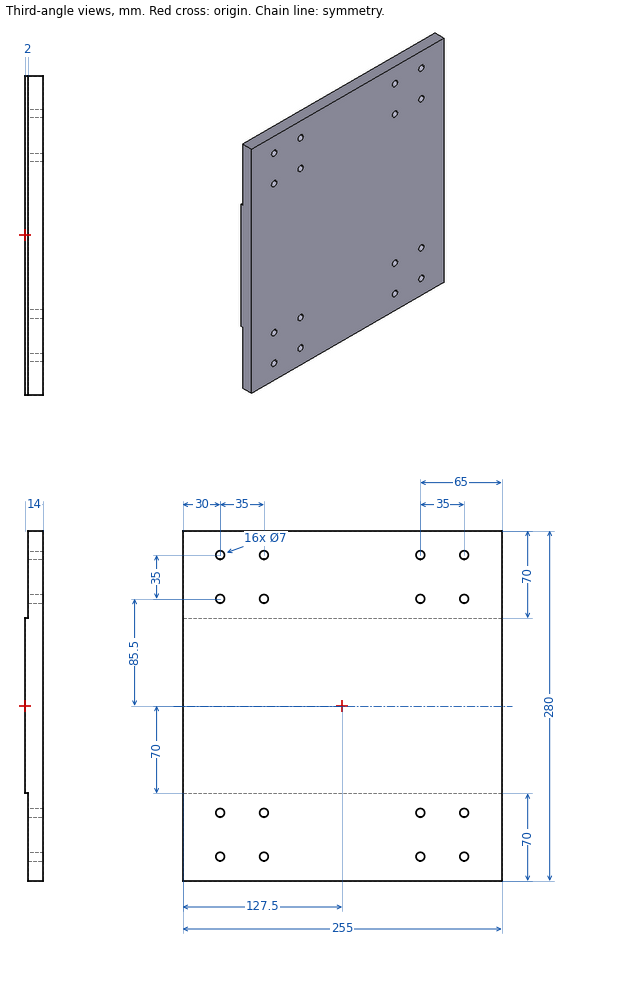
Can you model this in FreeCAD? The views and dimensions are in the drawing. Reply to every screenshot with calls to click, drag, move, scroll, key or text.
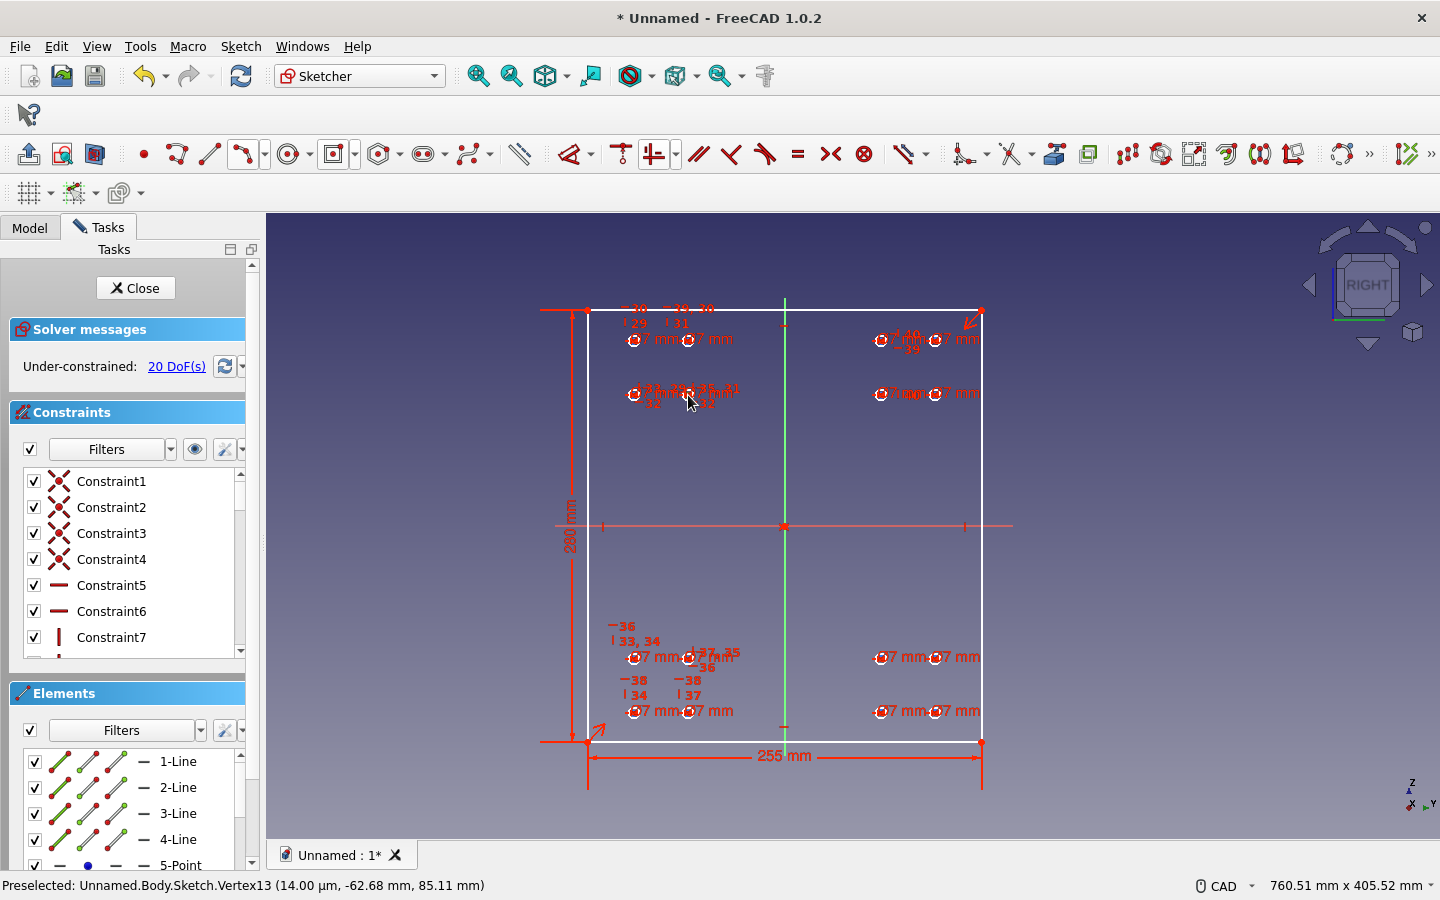
click(881, 395)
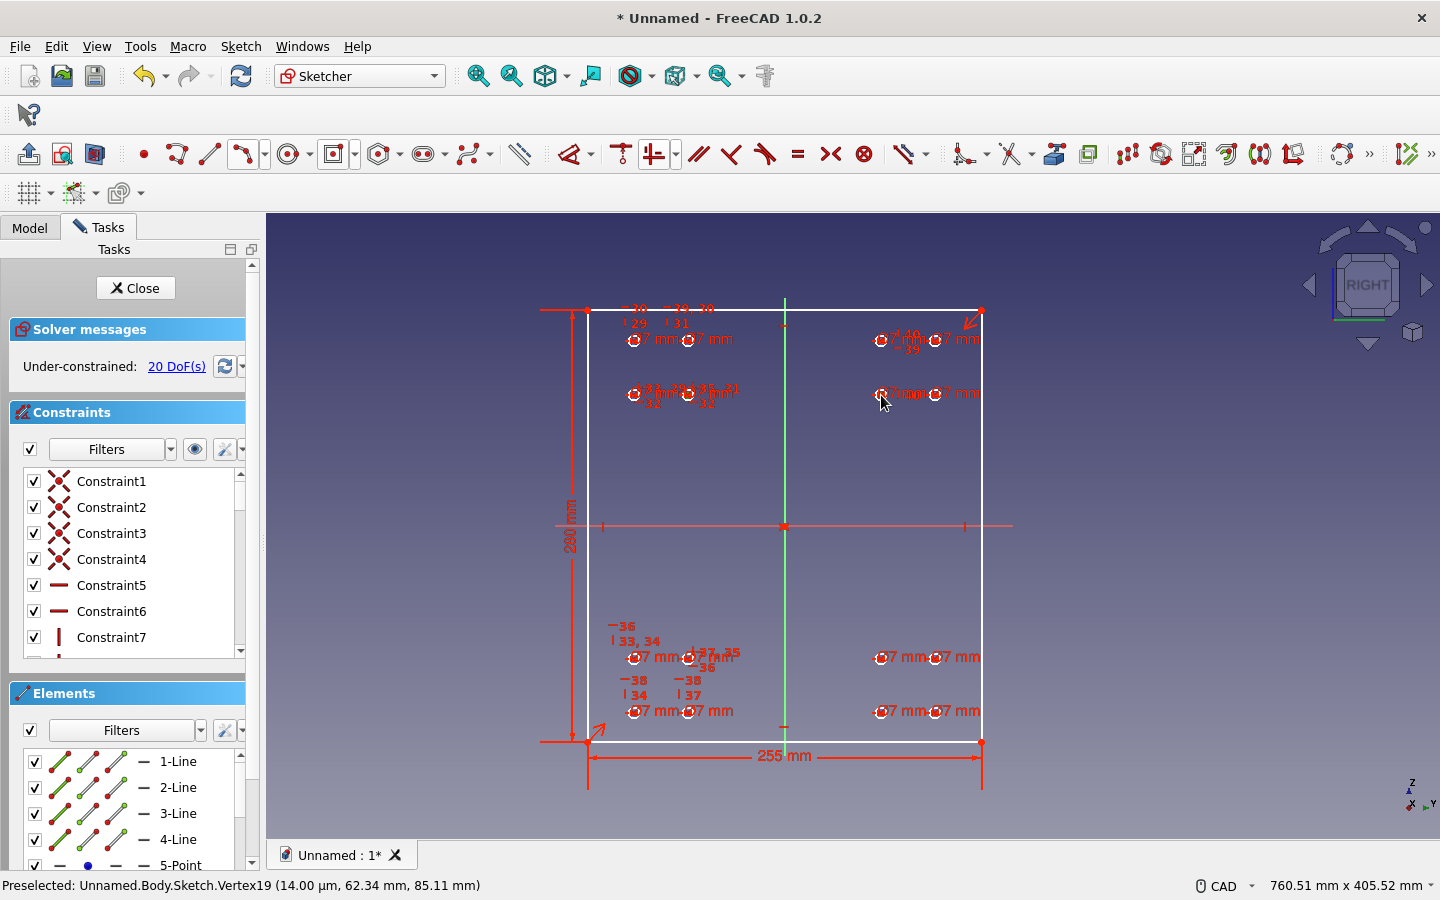
click(676, 154)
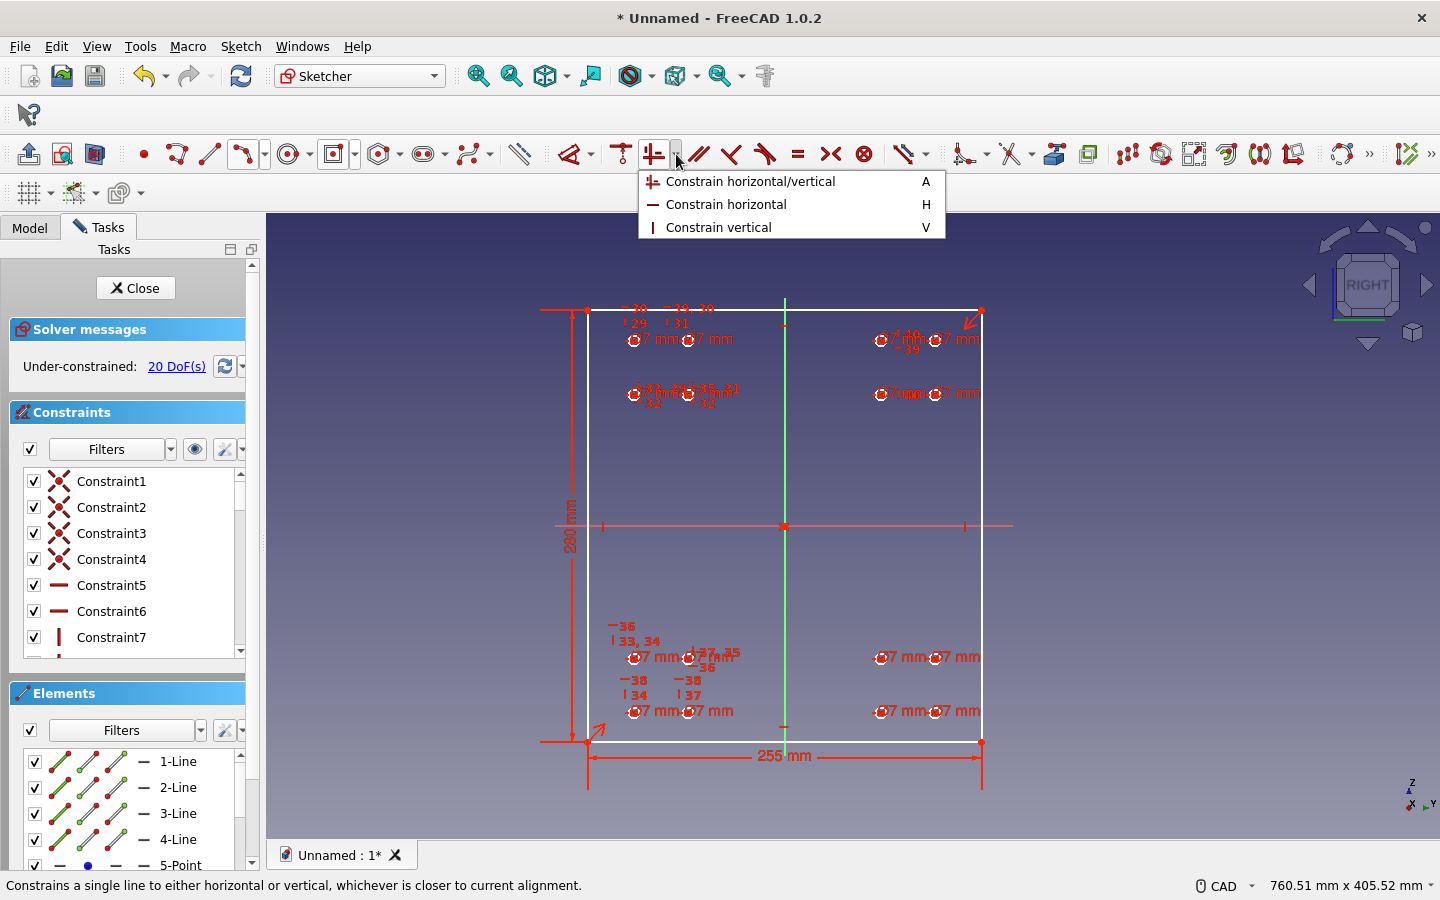
click(792, 204)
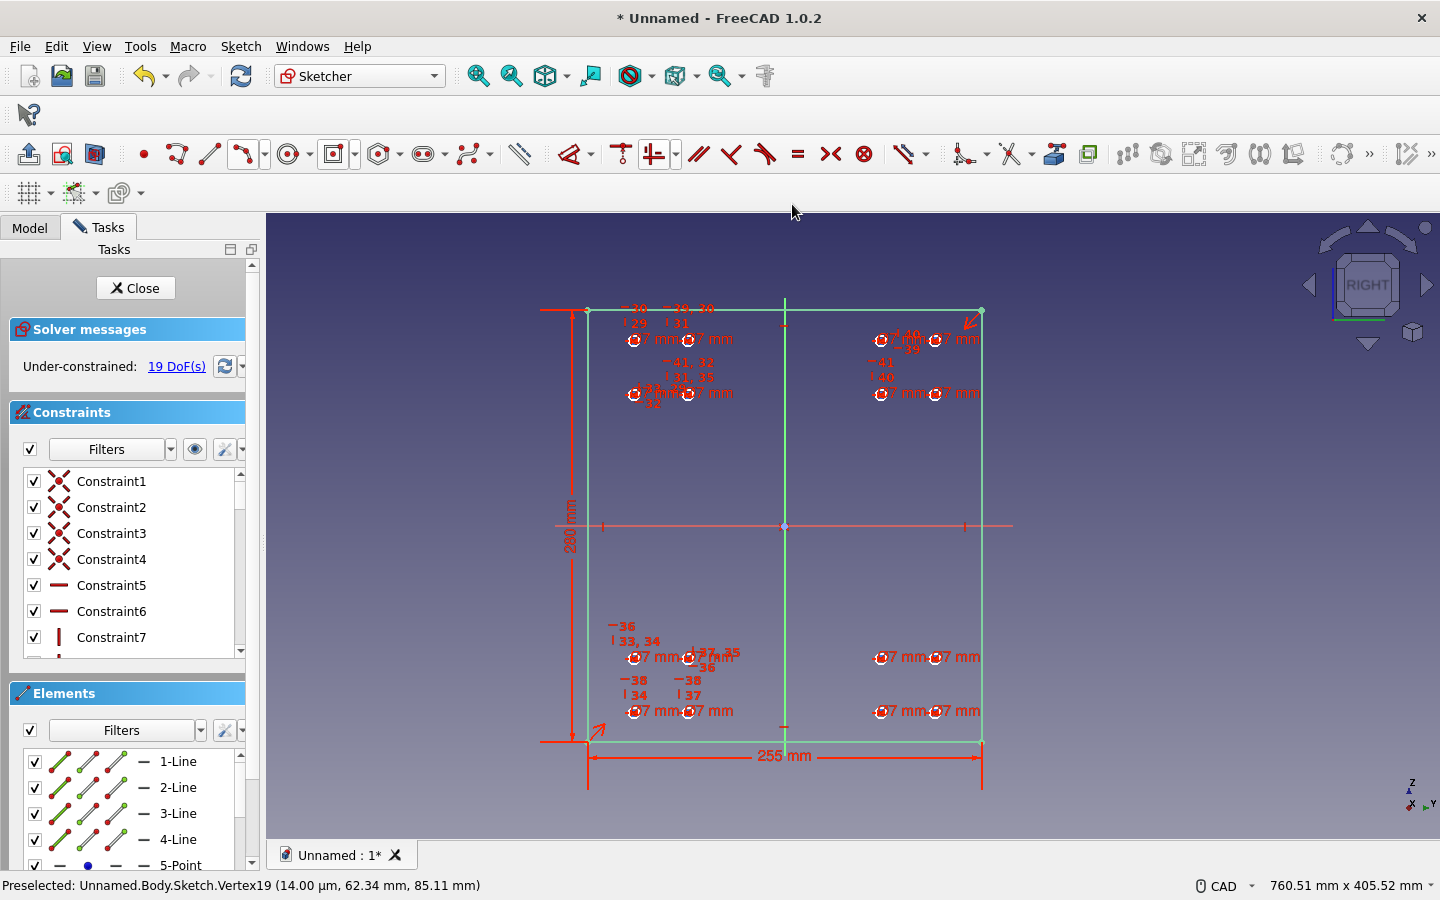
click(881, 341)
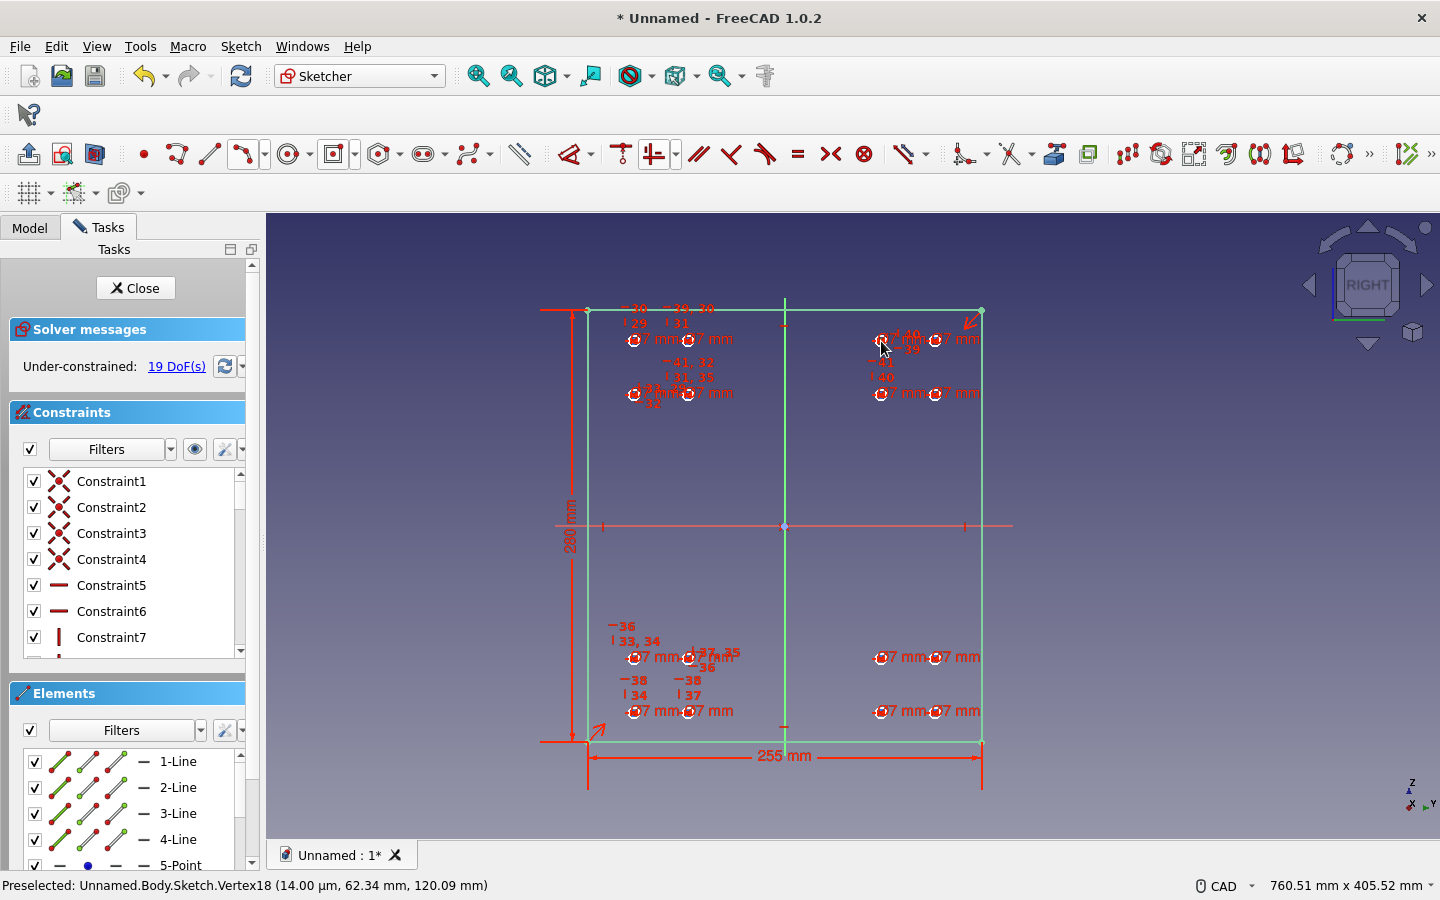
click(935, 341)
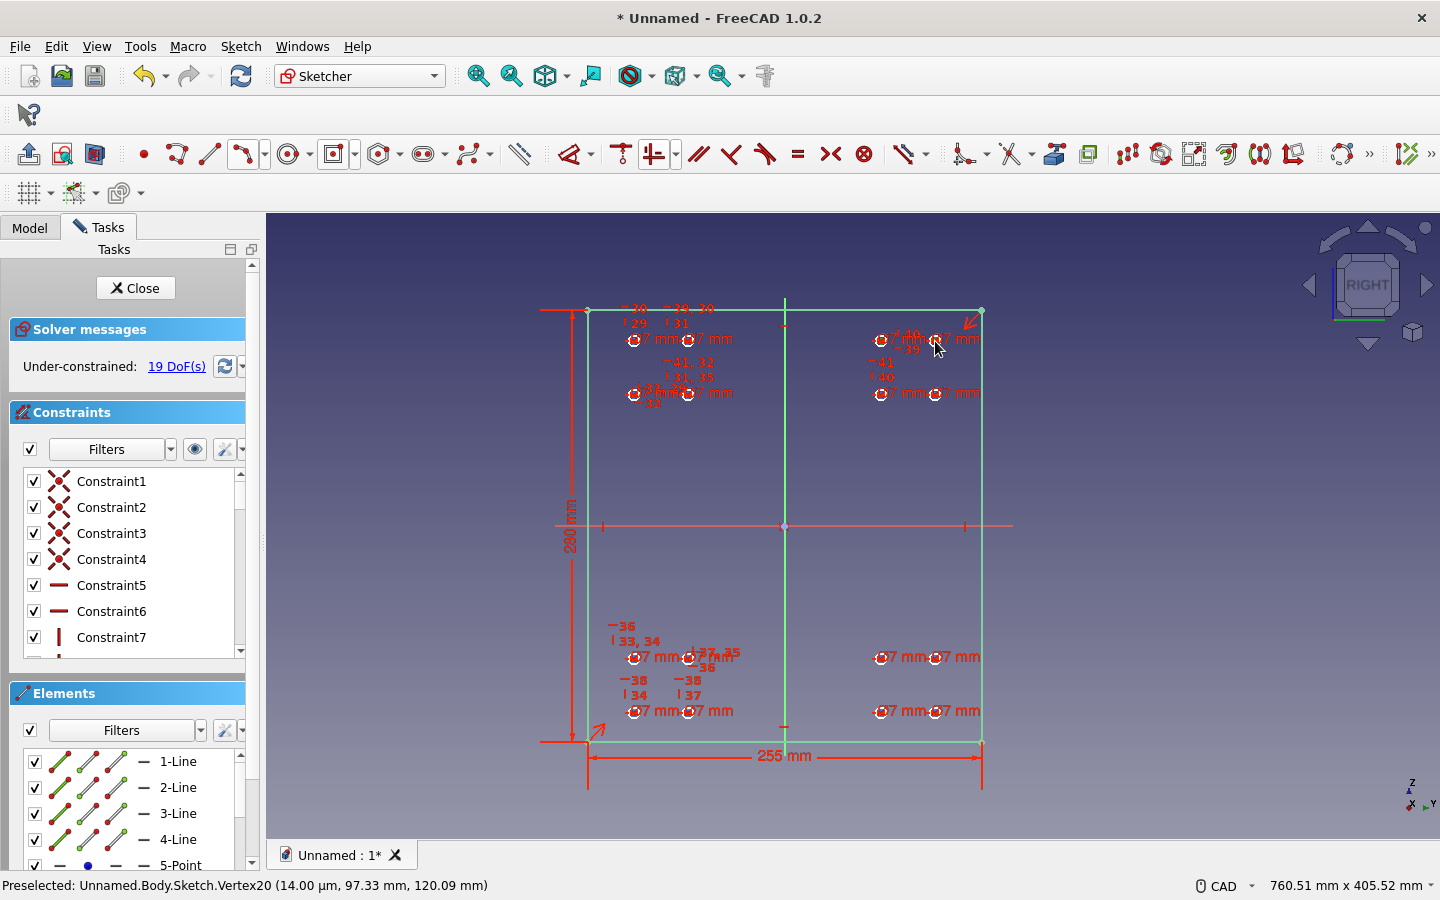
click(676, 154)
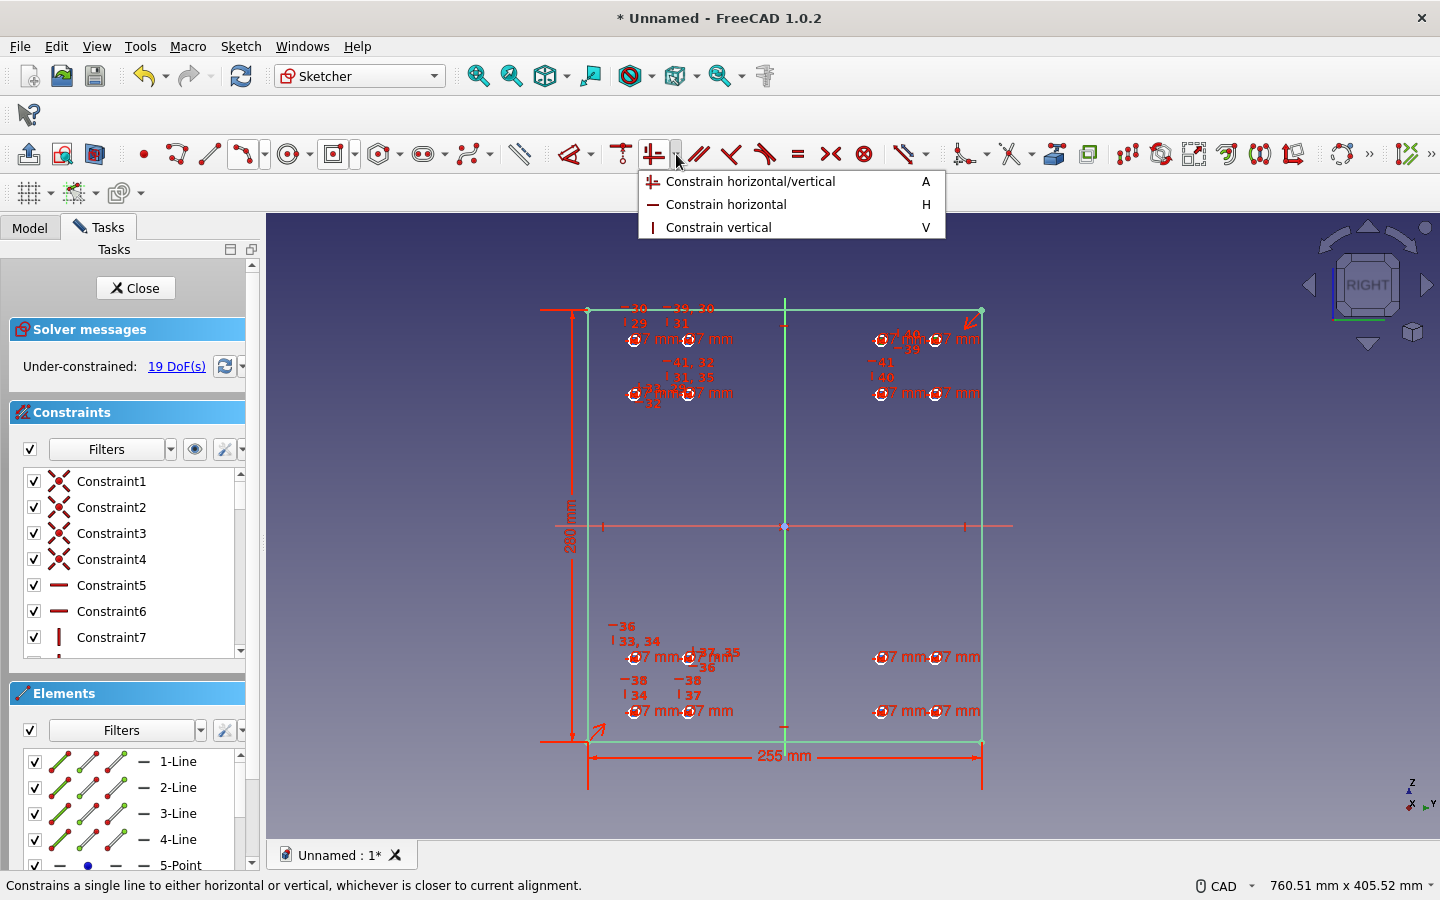
click(792, 204)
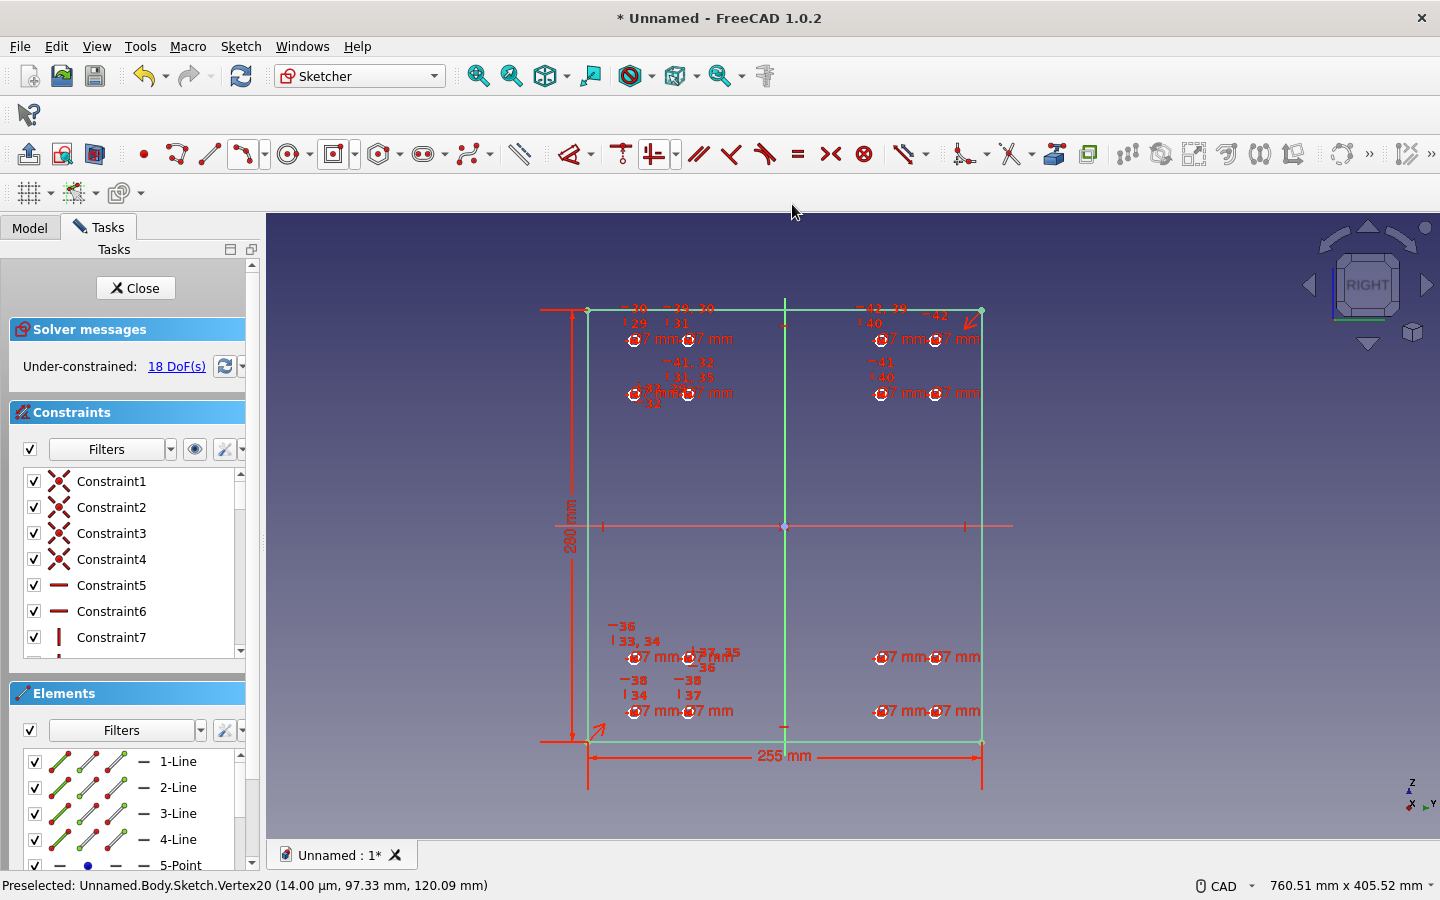
click(935, 341)